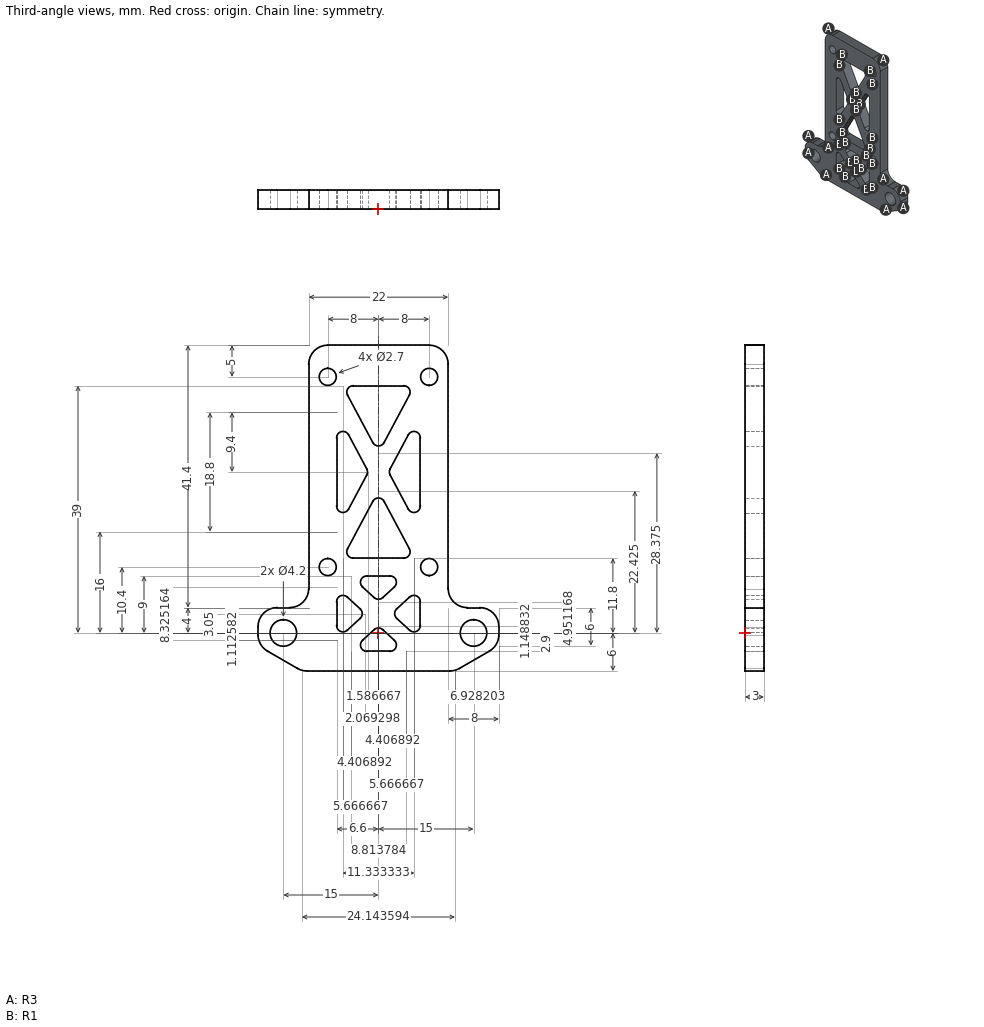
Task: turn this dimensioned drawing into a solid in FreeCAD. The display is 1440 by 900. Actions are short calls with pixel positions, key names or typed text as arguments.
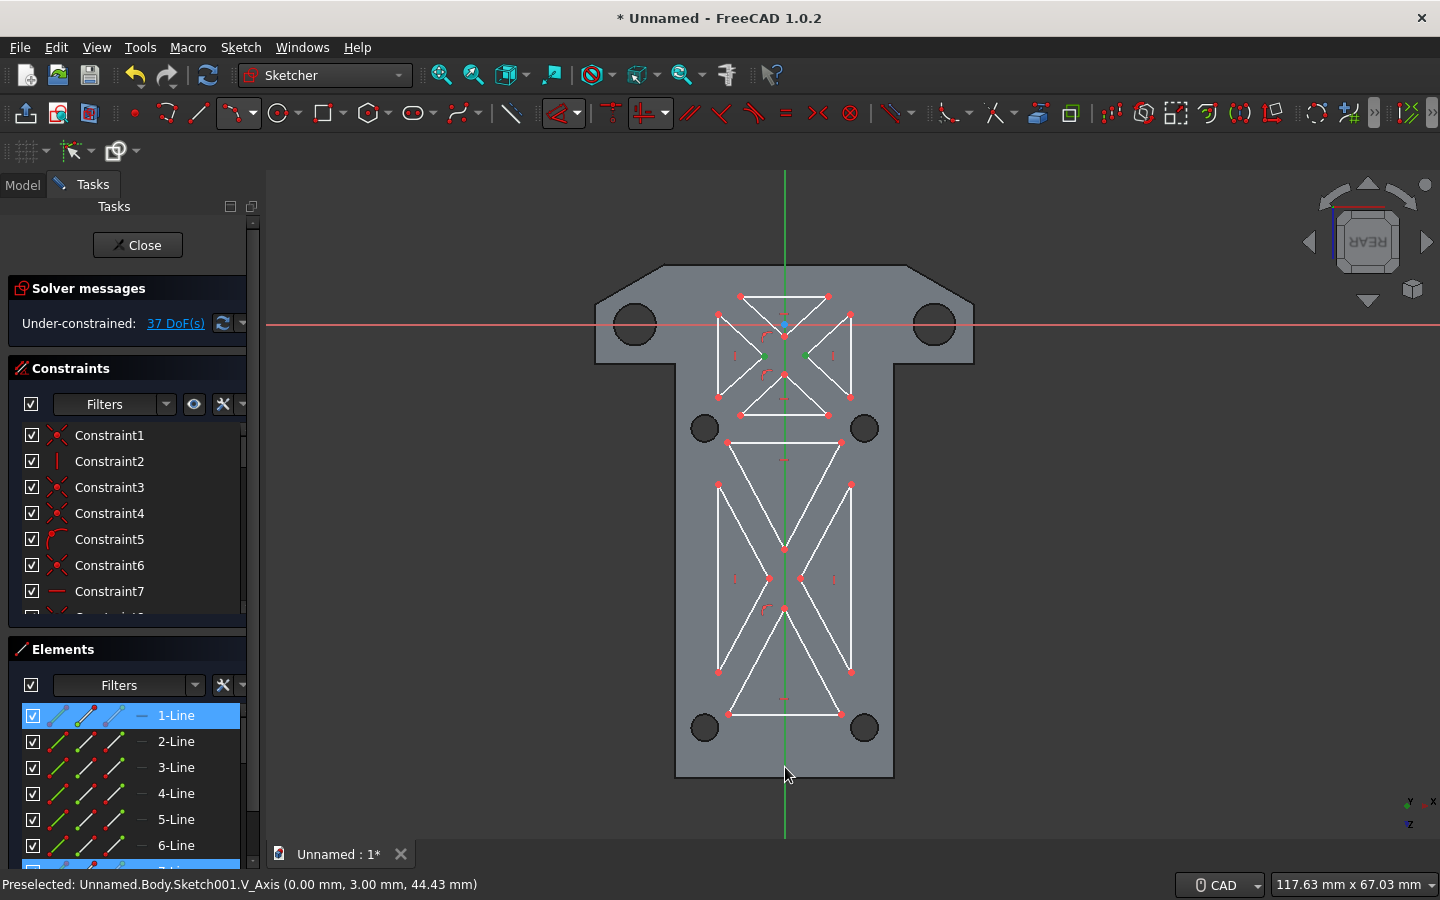
click(818, 114)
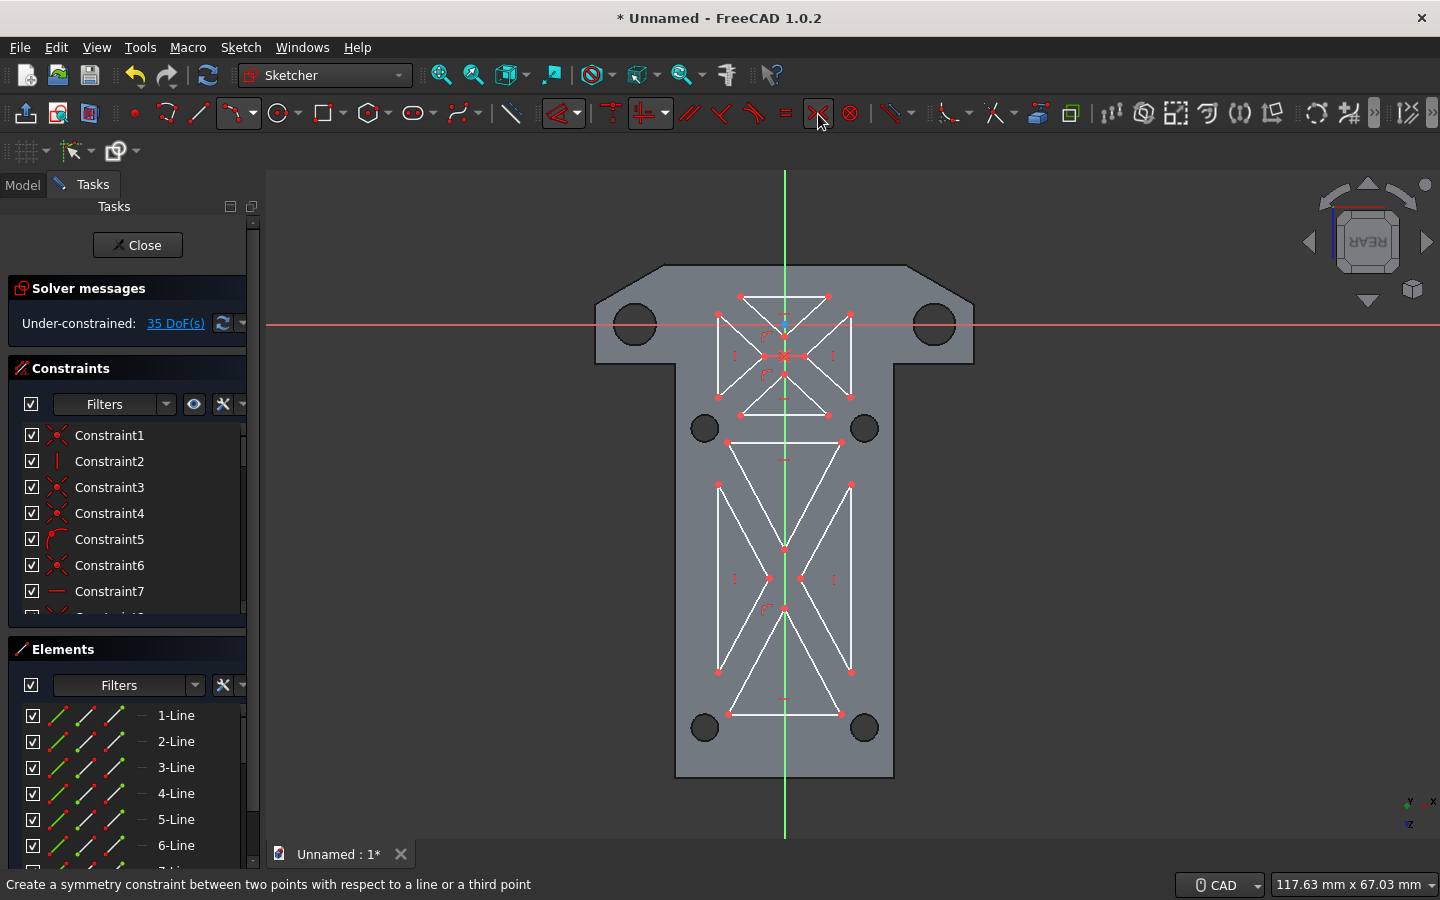
click(718, 397)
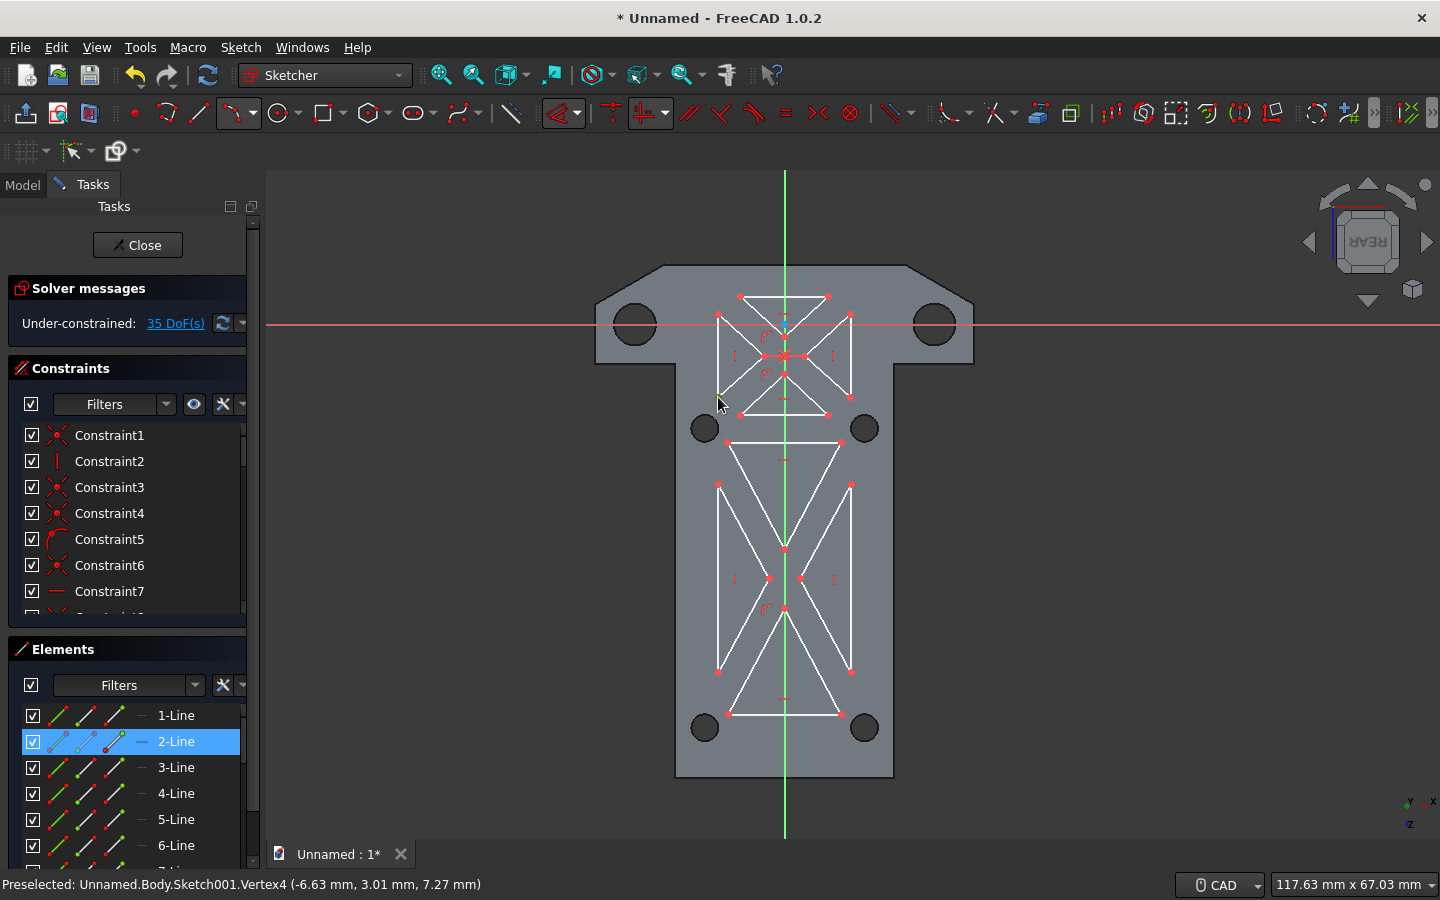
click(851, 397)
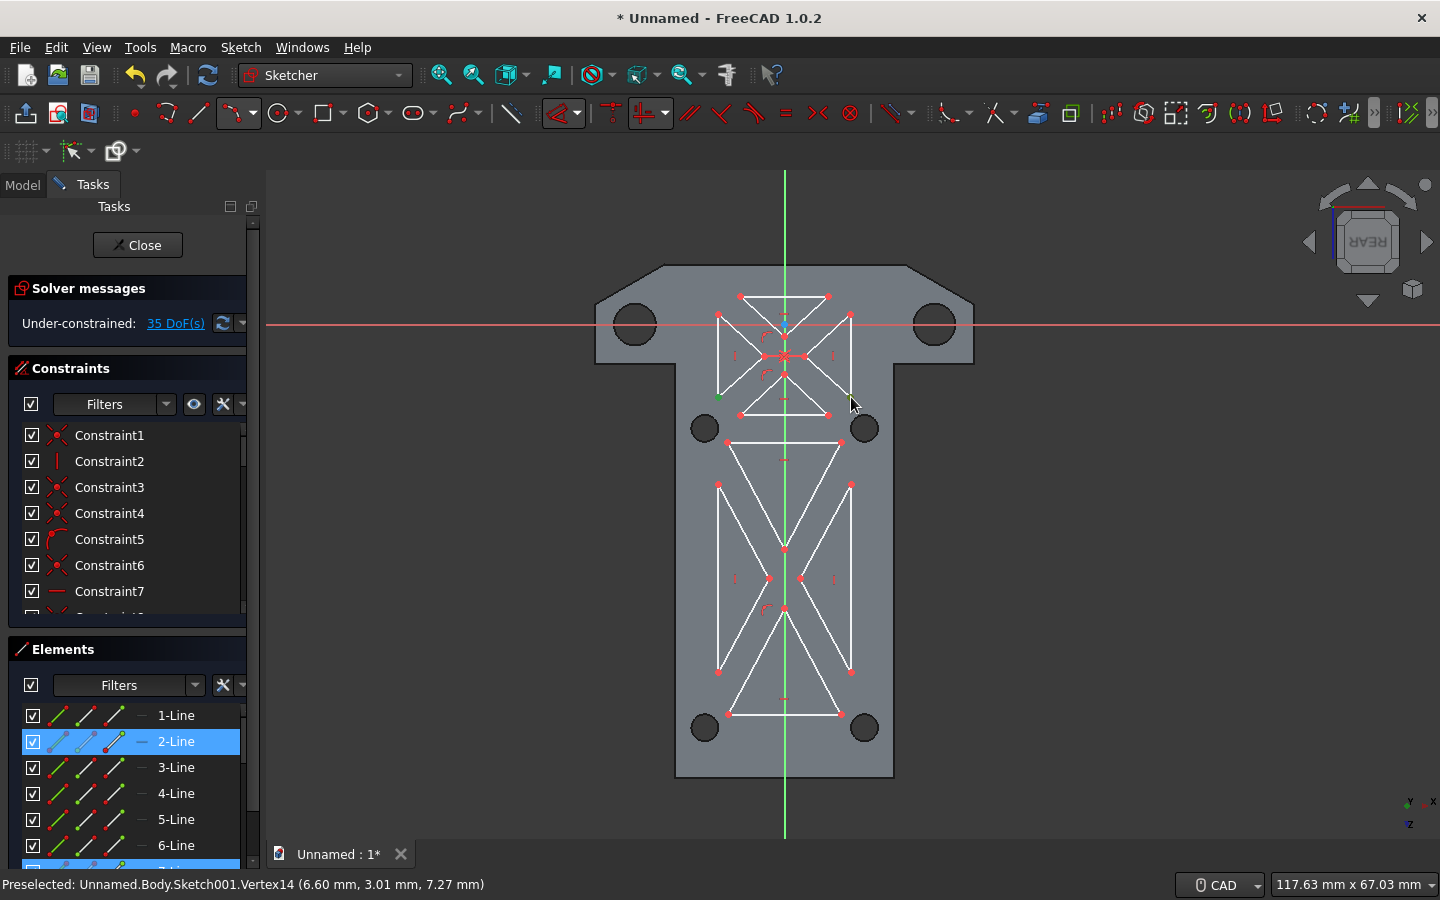
click(785, 767)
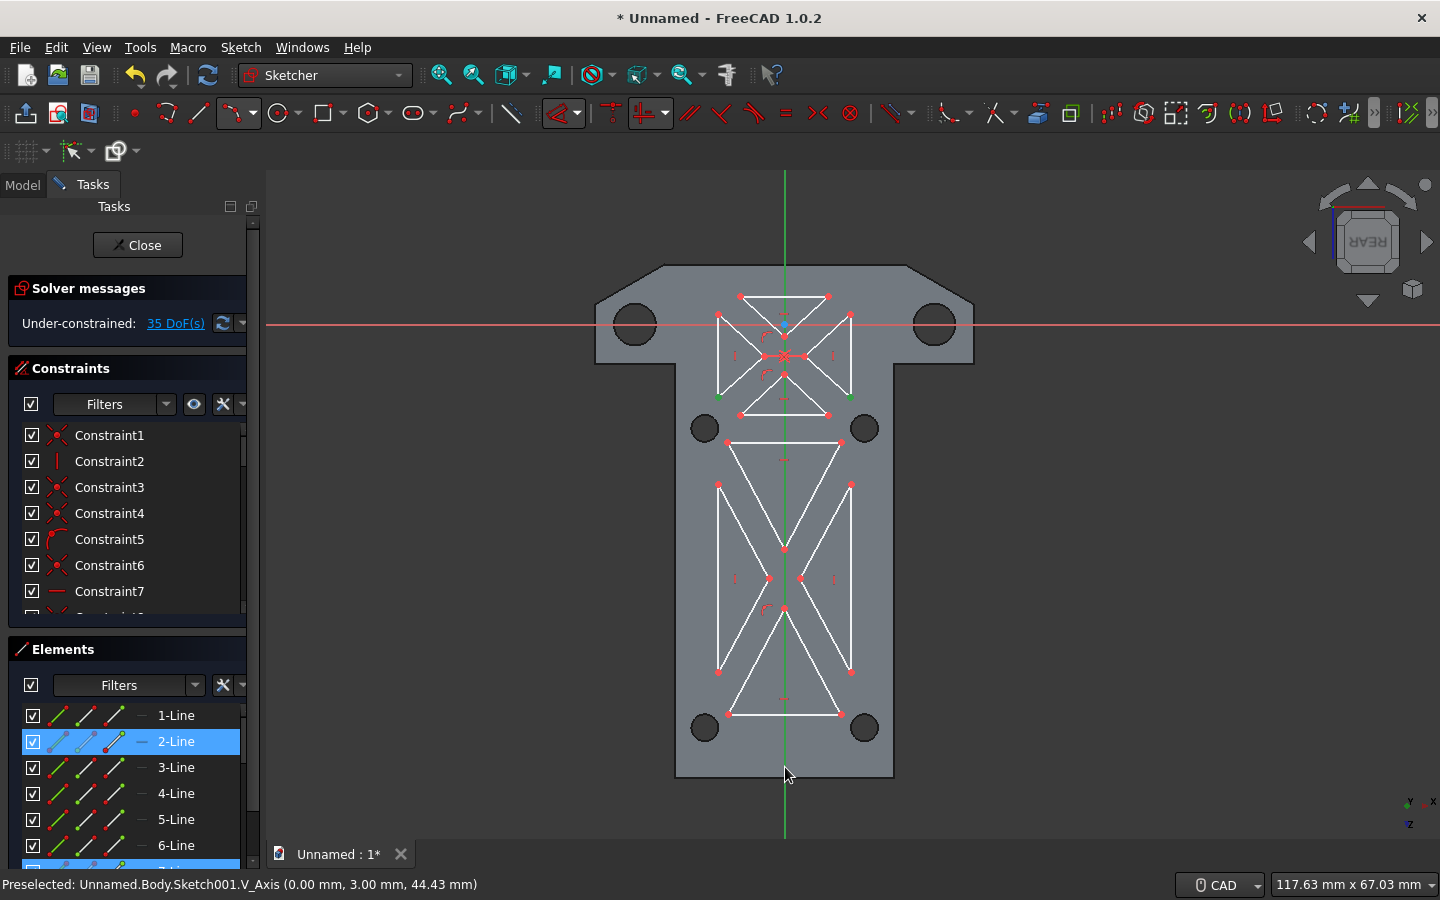
click(818, 114)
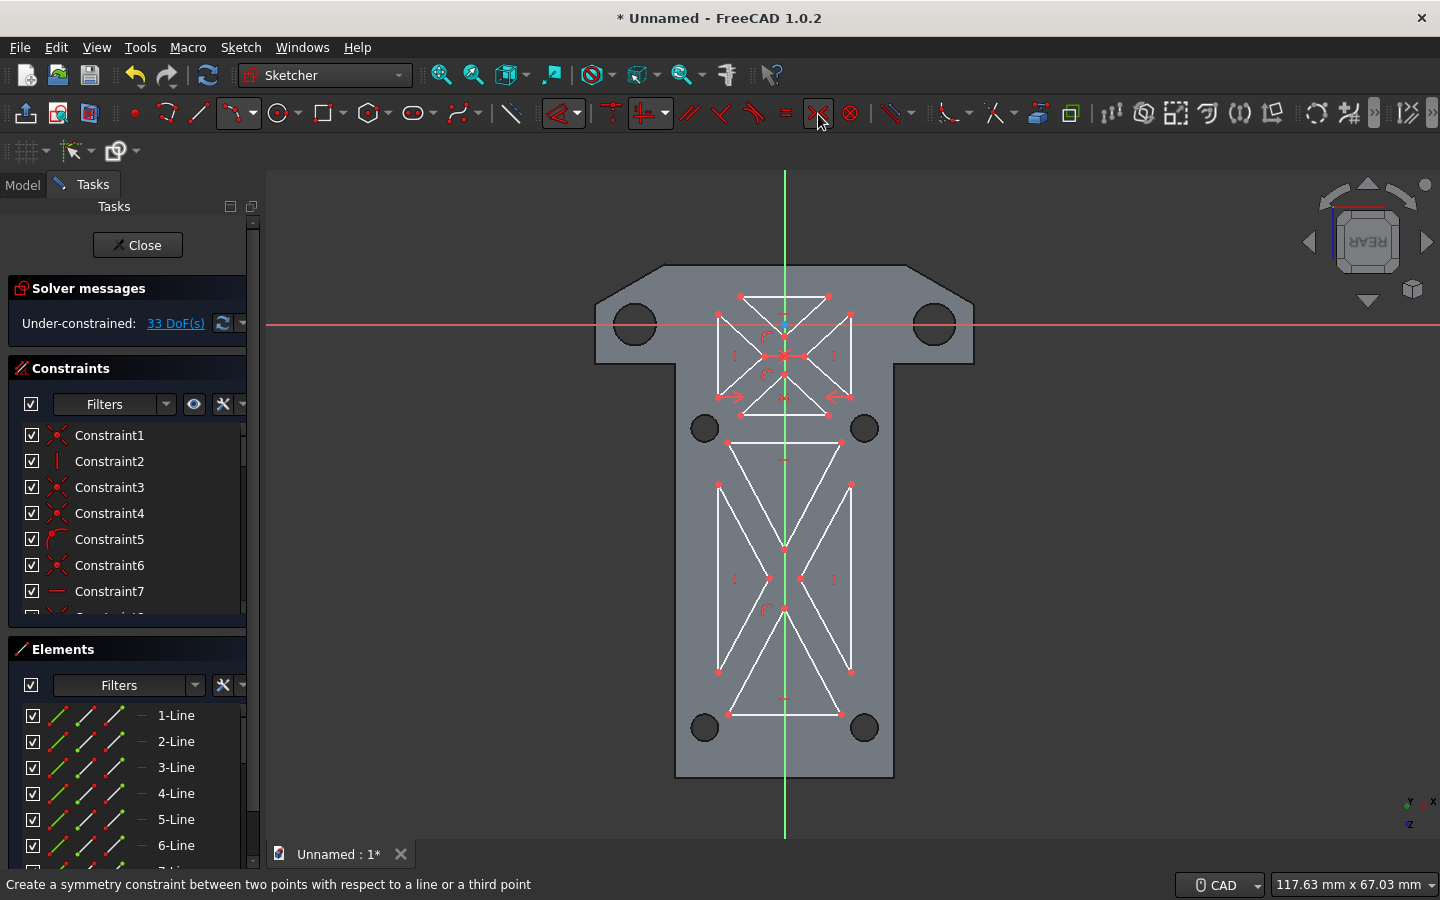
click(718, 485)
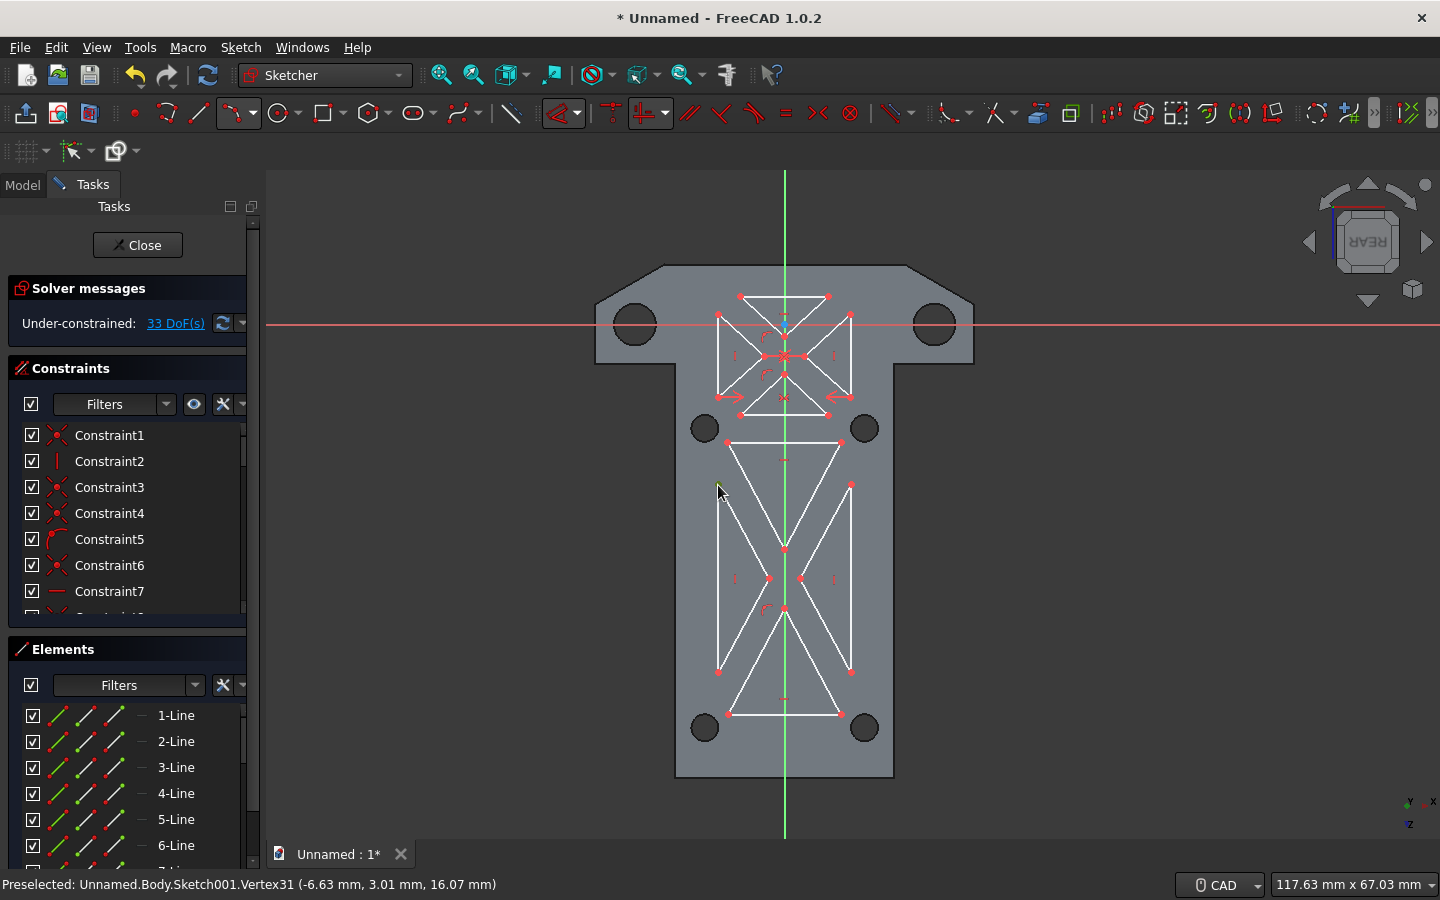
click(851, 485)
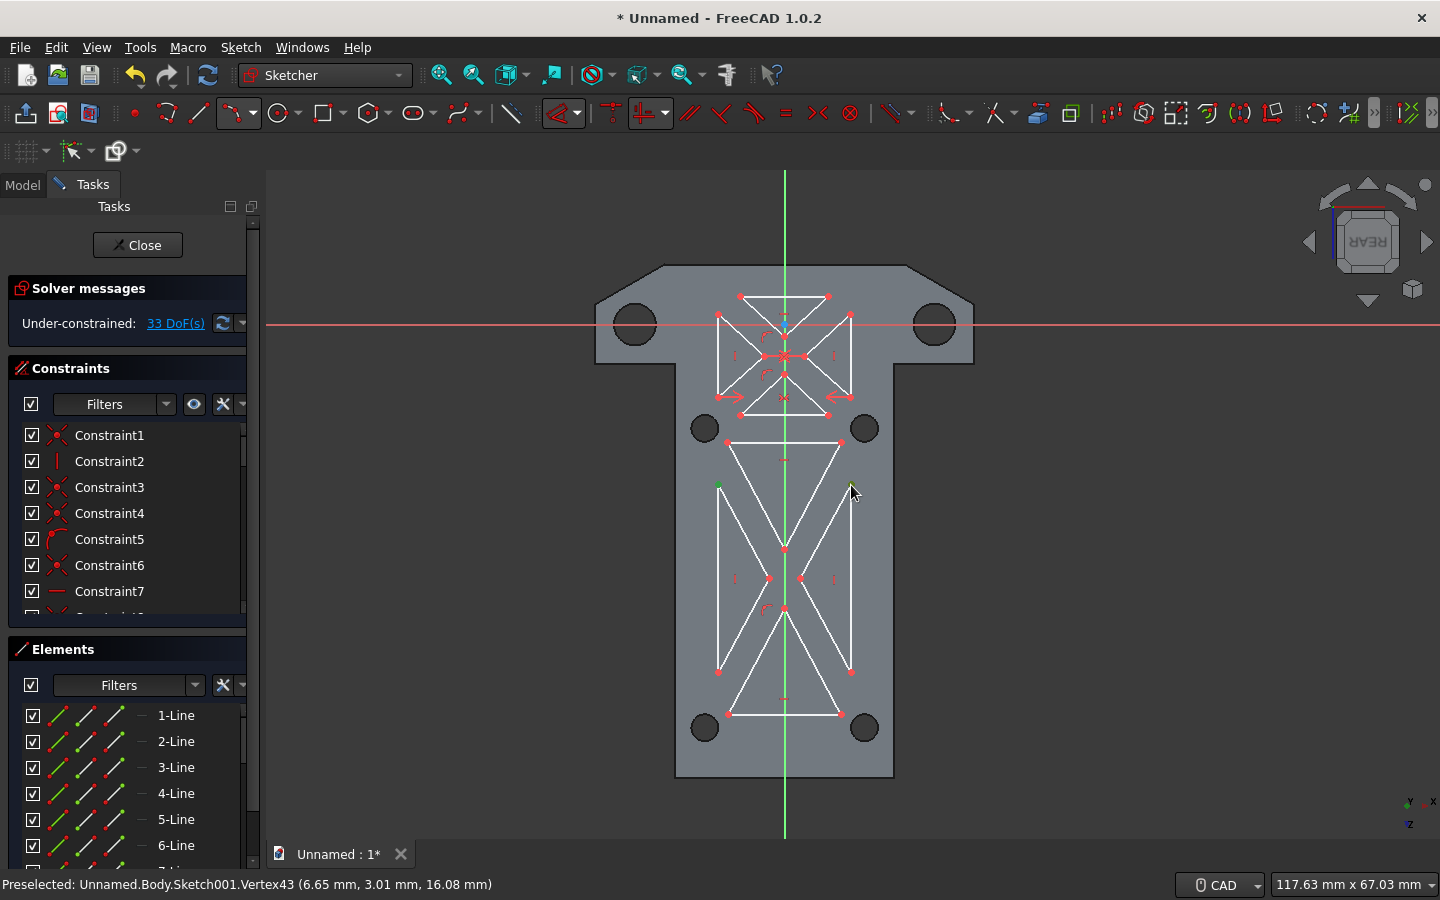
click(785, 767)